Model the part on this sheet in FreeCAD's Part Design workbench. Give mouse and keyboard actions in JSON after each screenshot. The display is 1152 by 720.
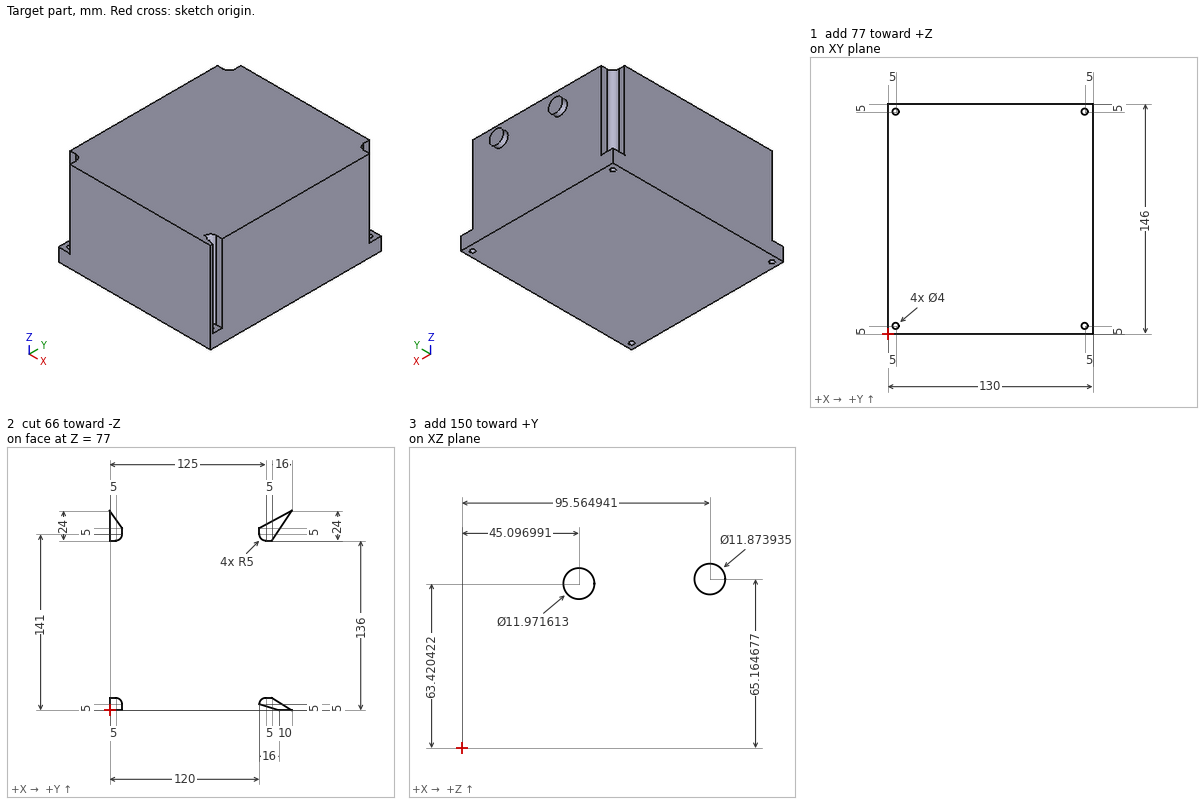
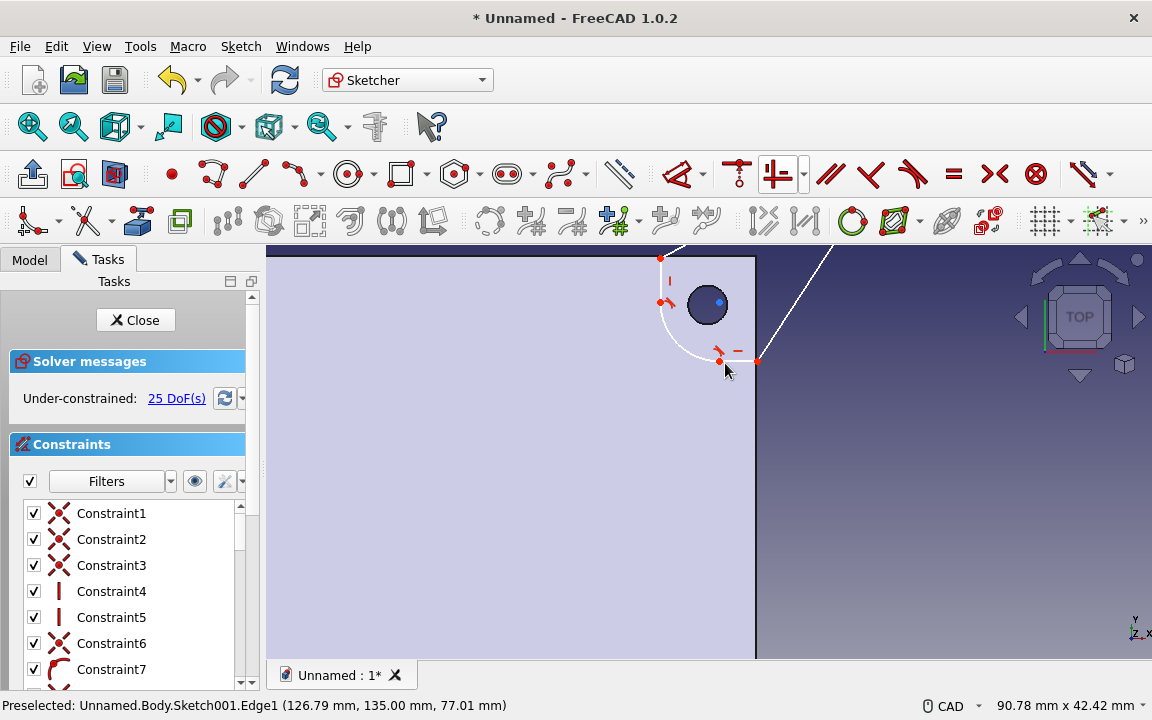
{"action": "scroll", "coordinate": [728, 363], "scroll_direction": "down", "scroll_amount": 9}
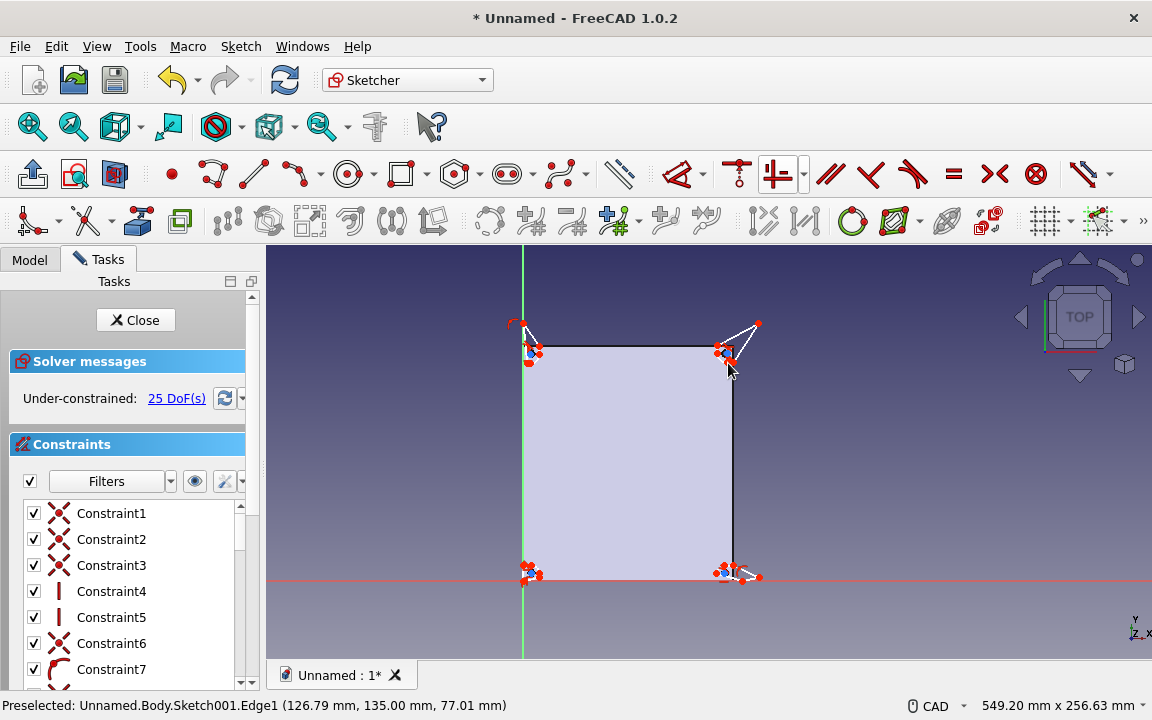
{"action": "scroll", "coordinate": [526, 352], "scroll_direction": "up", "scroll_amount": 9}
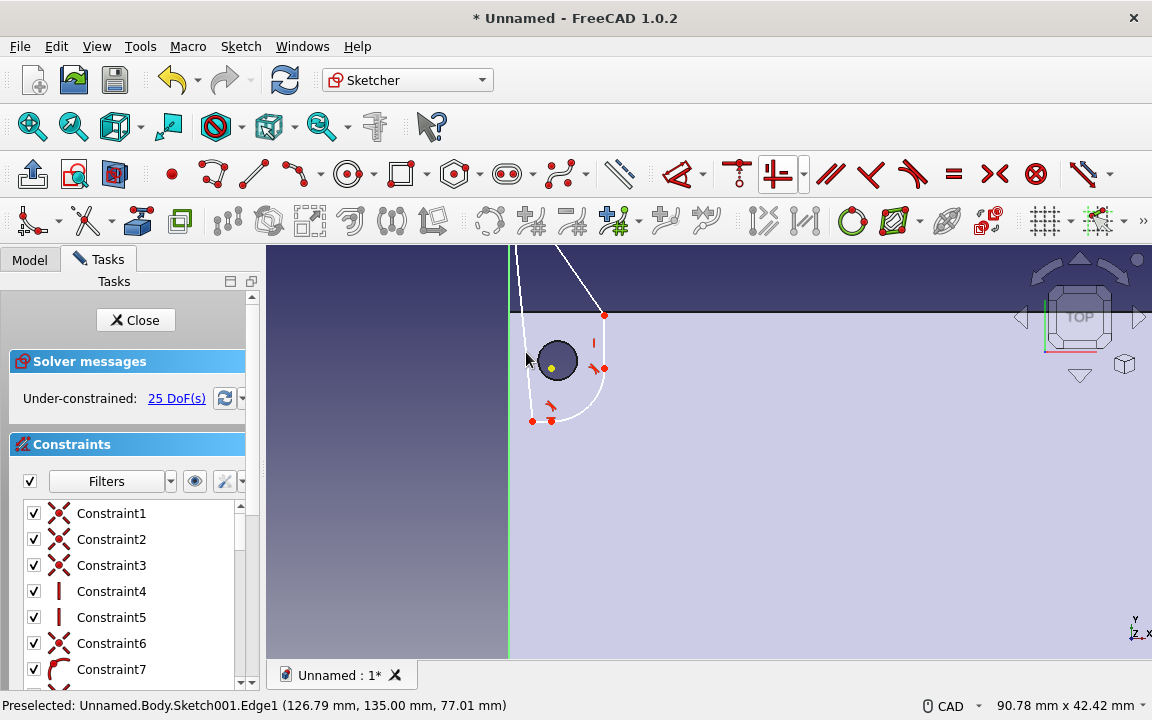
{"action": "left_click", "coordinate": [526, 348]}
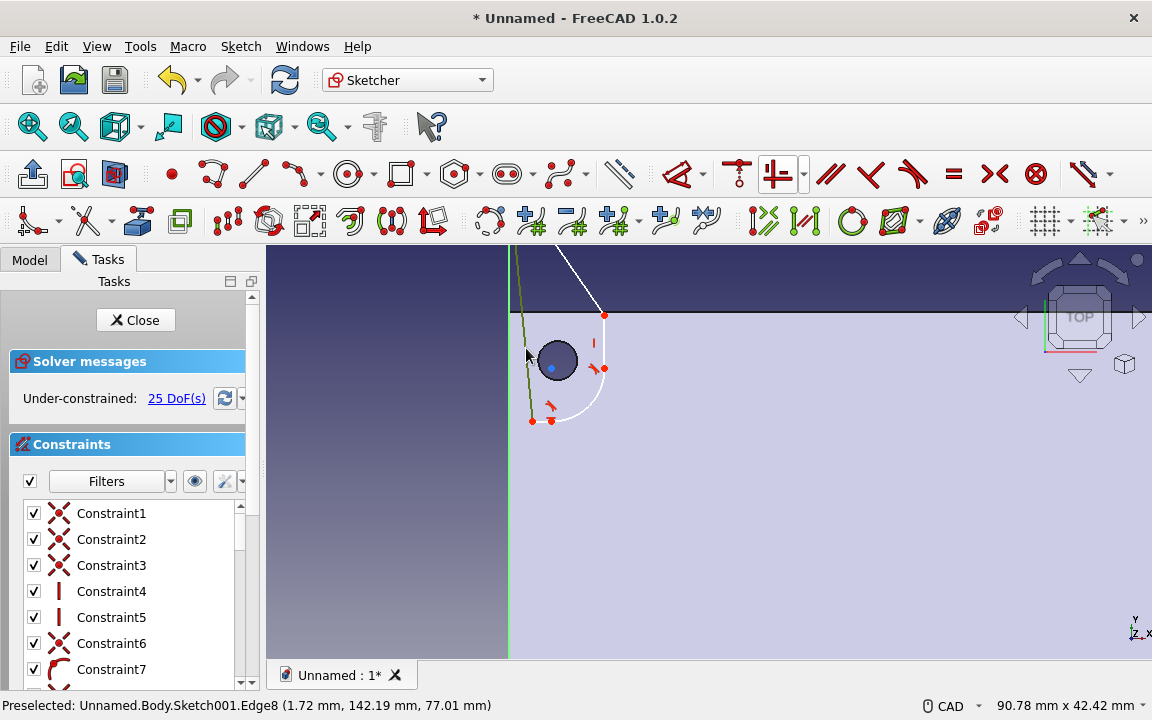
{"action": "left_click", "coordinate": [804, 174]}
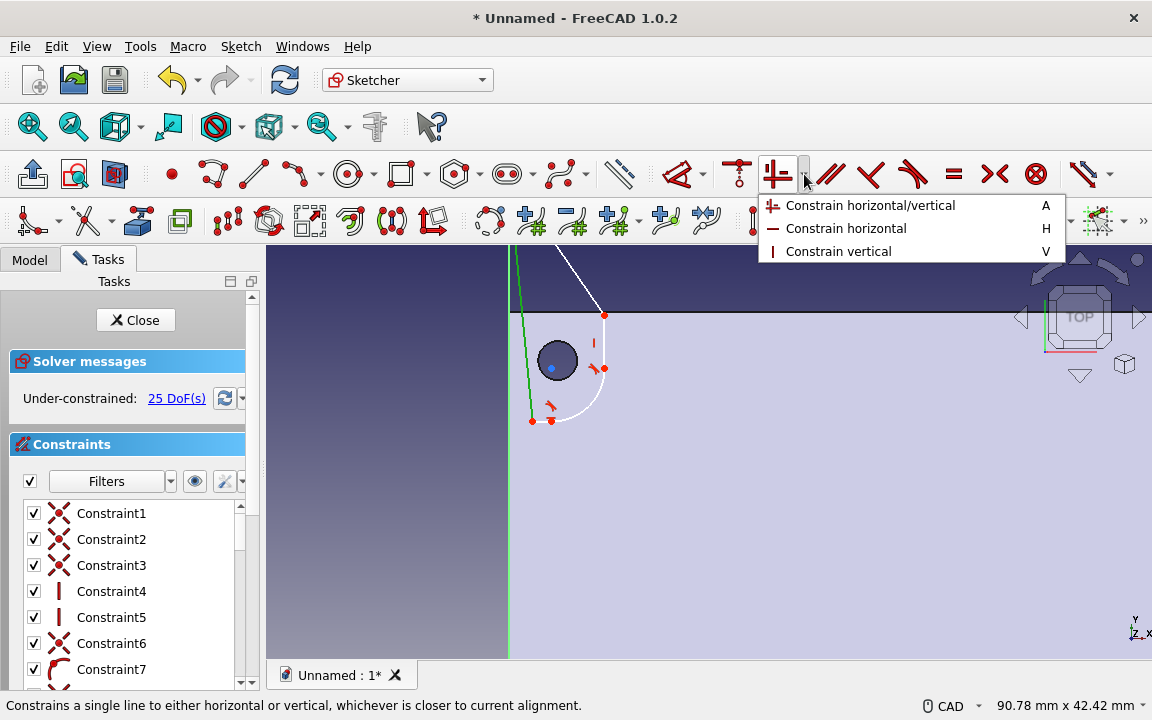
{"action": "left_click", "coordinate": [912, 252]}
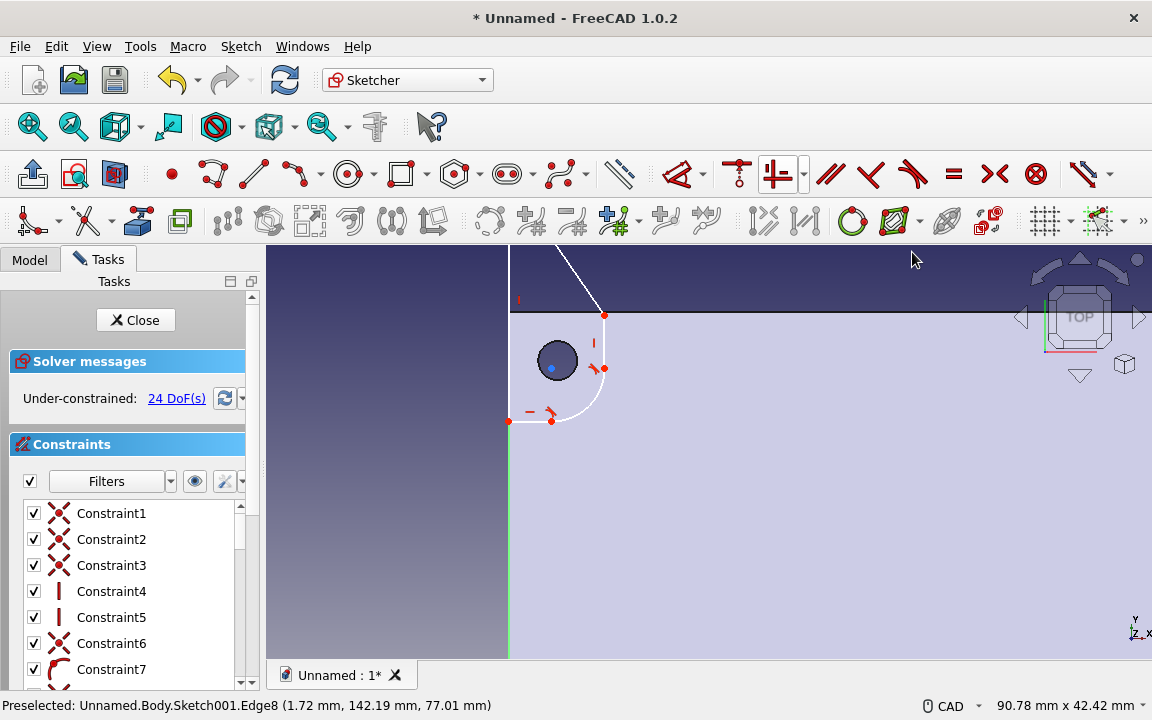
{"action": "scroll", "coordinate": [525, 352], "scroll_direction": "down", "scroll_amount": 9}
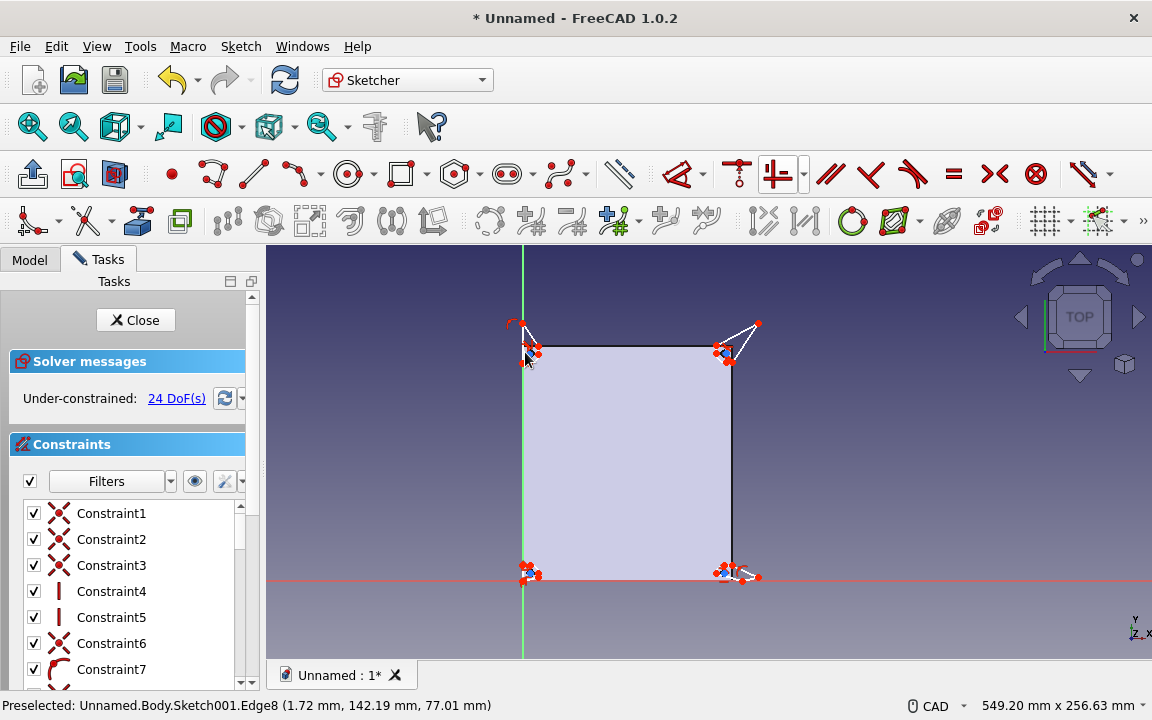
{"action": "scroll", "coordinate": [534, 579], "scroll_direction": "up", "scroll_amount": 9}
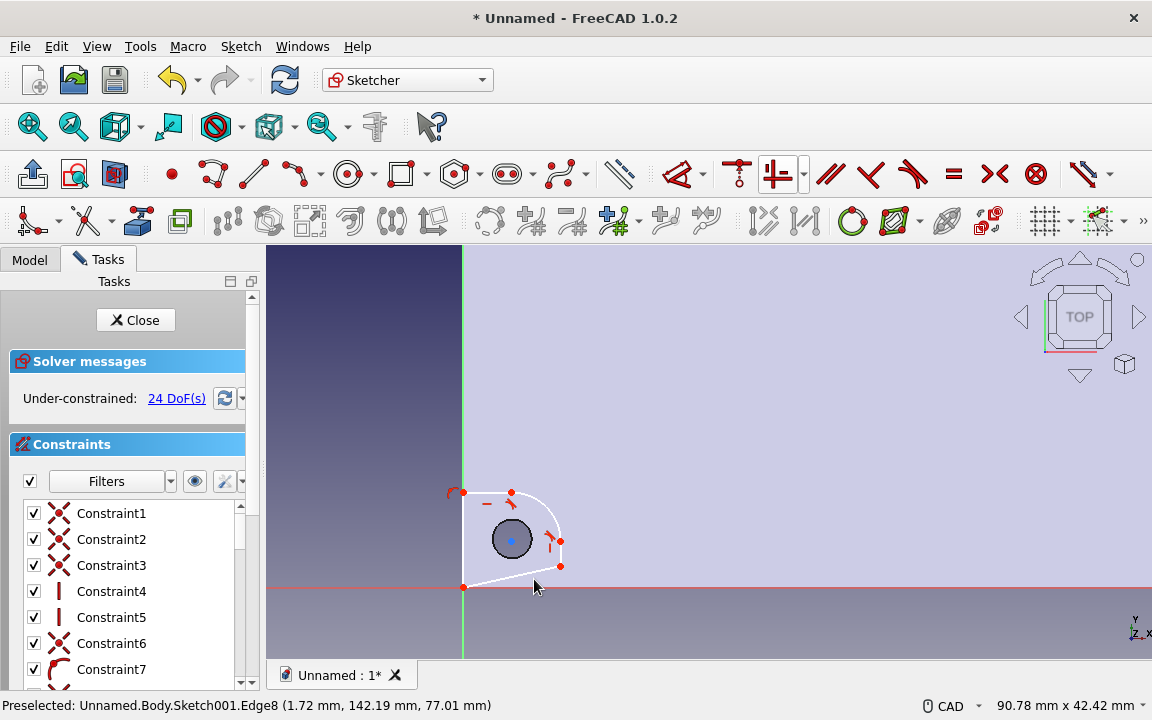
{"action": "left_click", "coordinate": [531, 573]}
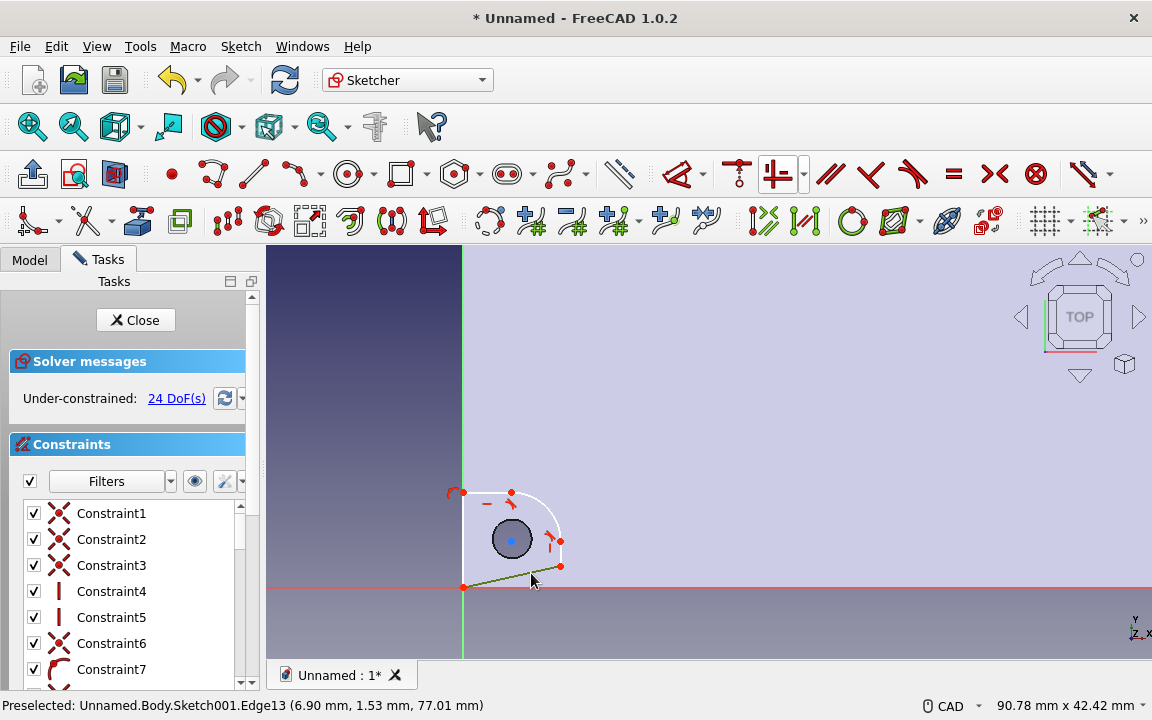
{"action": "key", "text": "h"}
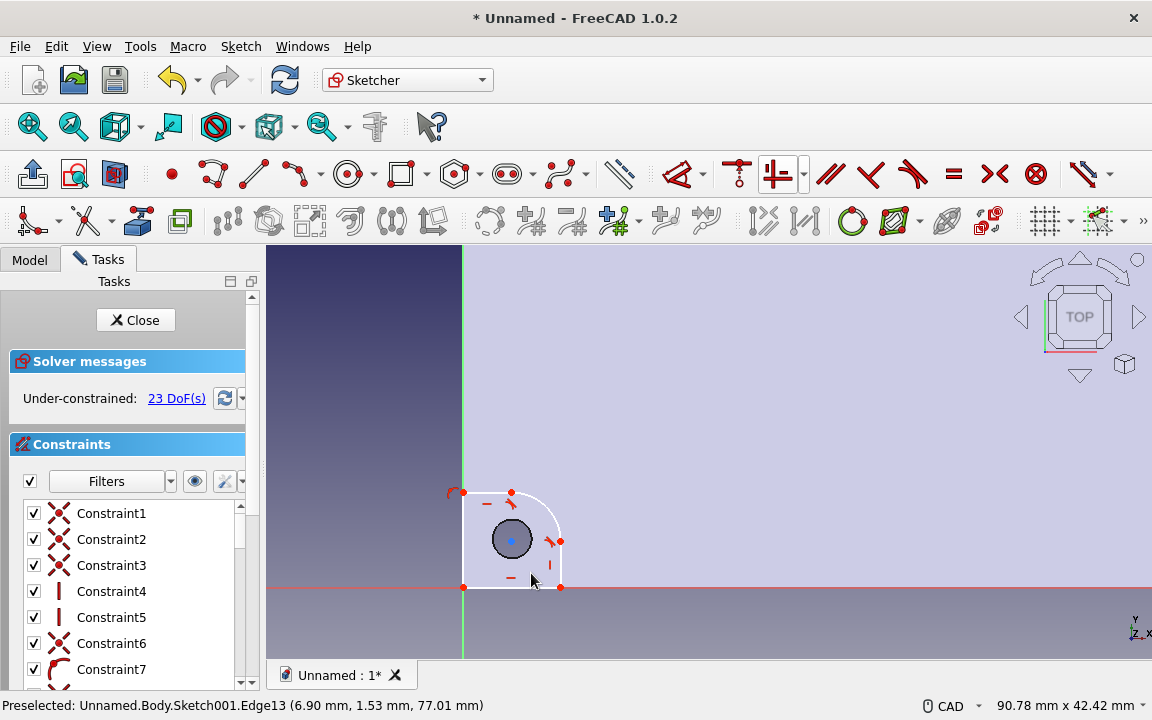
{"action": "scroll", "coordinate": [534, 580], "scroll_direction": "down", "scroll_amount": 9}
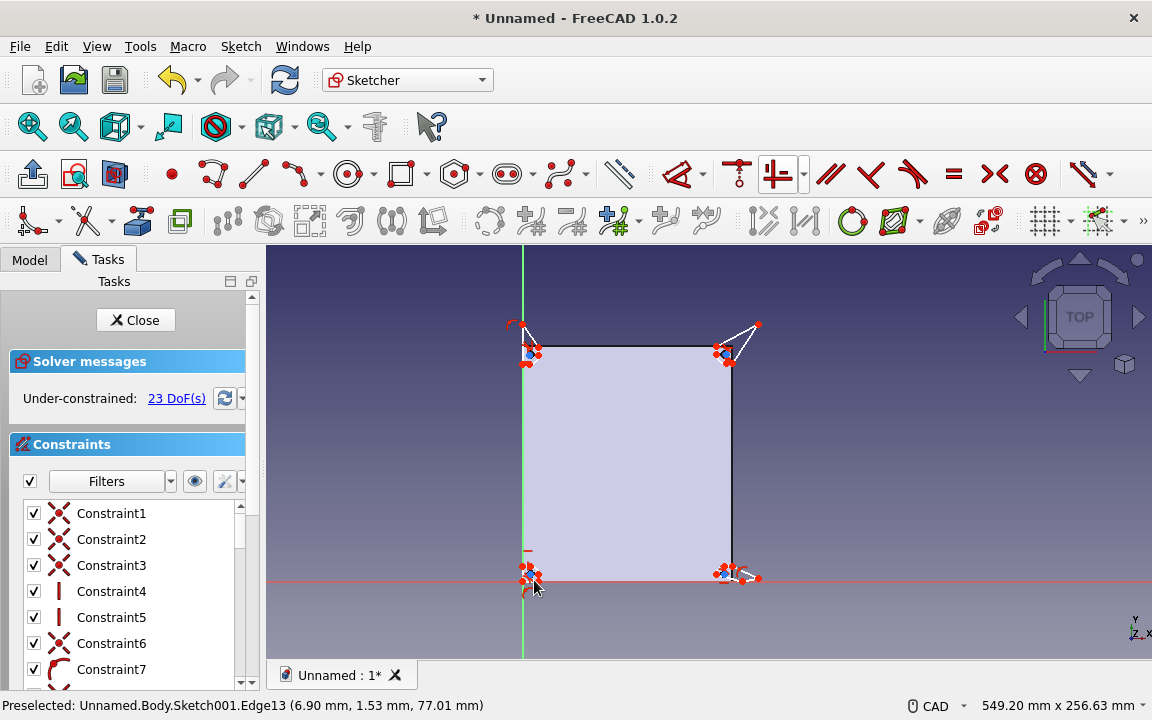
{"action": "scroll", "coordinate": [753, 580], "scroll_direction": "up", "scroll_amount": 9}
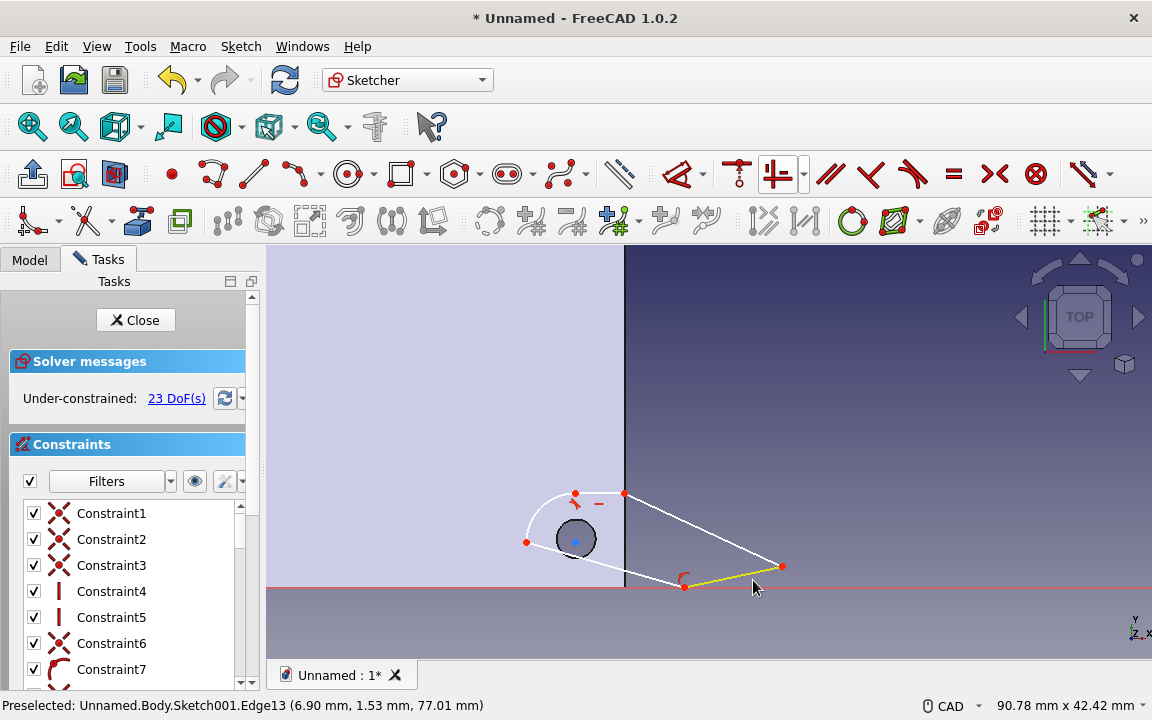
{"action": "left_click", "coordinate": [753, 573]}